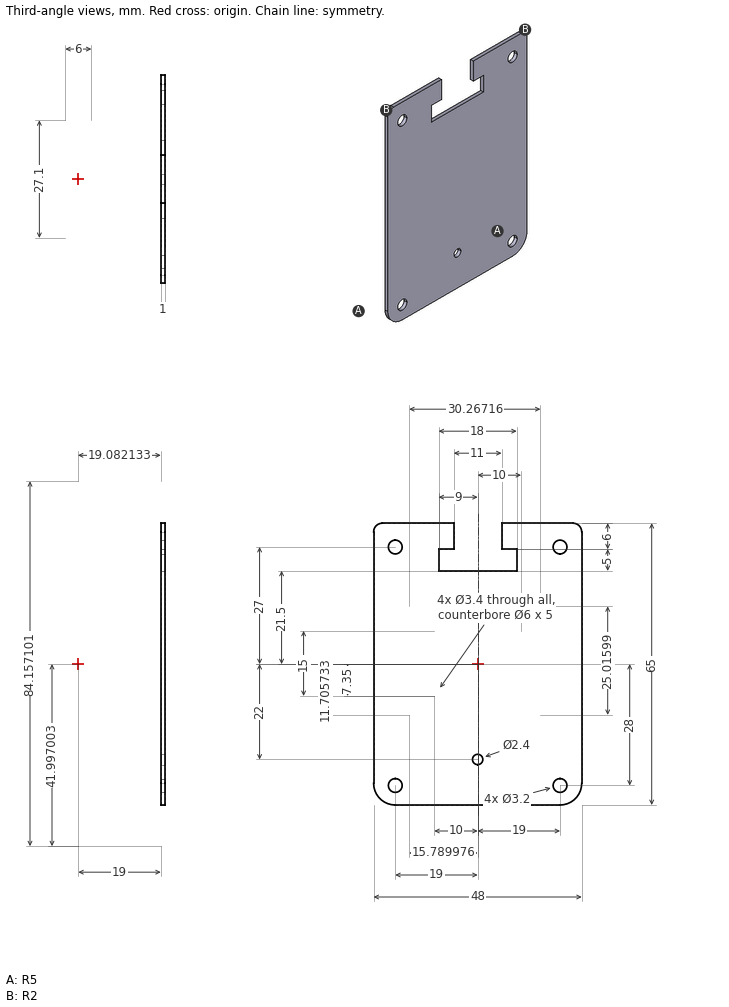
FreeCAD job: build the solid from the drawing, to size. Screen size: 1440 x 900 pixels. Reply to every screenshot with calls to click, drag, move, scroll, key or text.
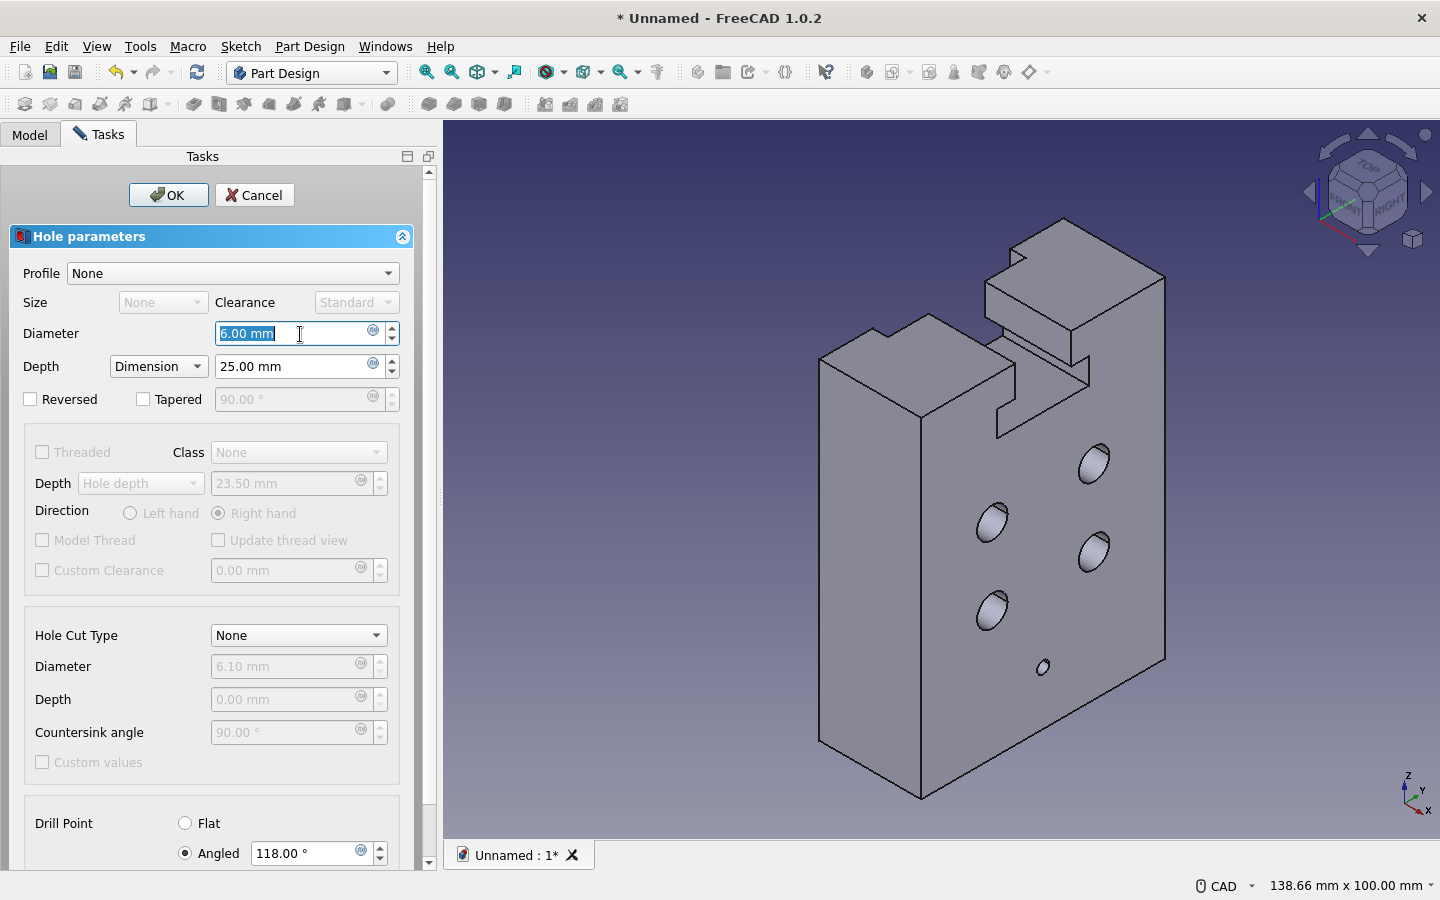
text(3.4)
key(Tab)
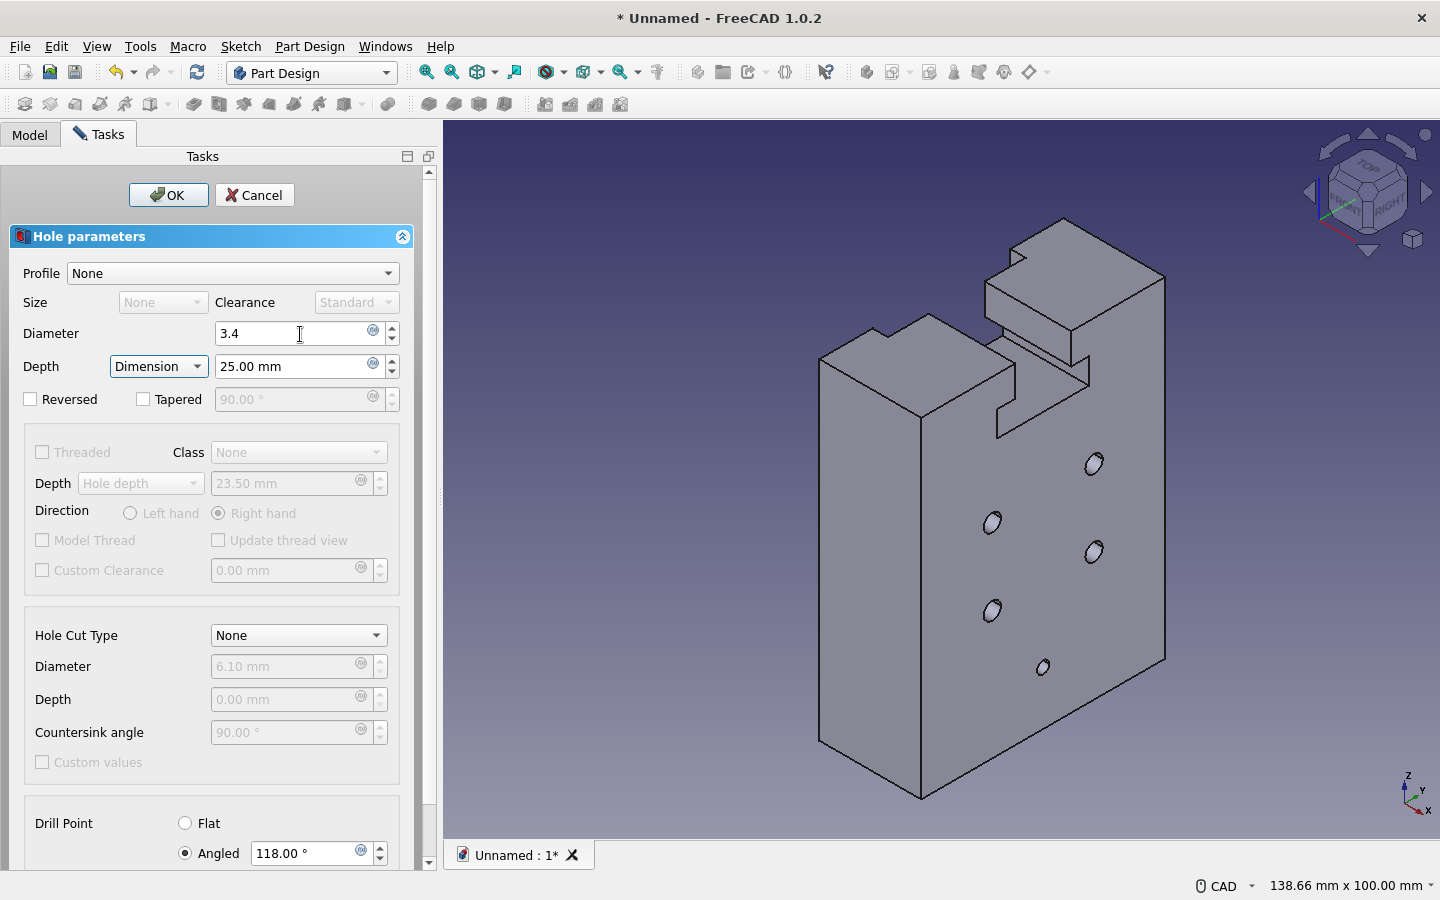
click(160, 366)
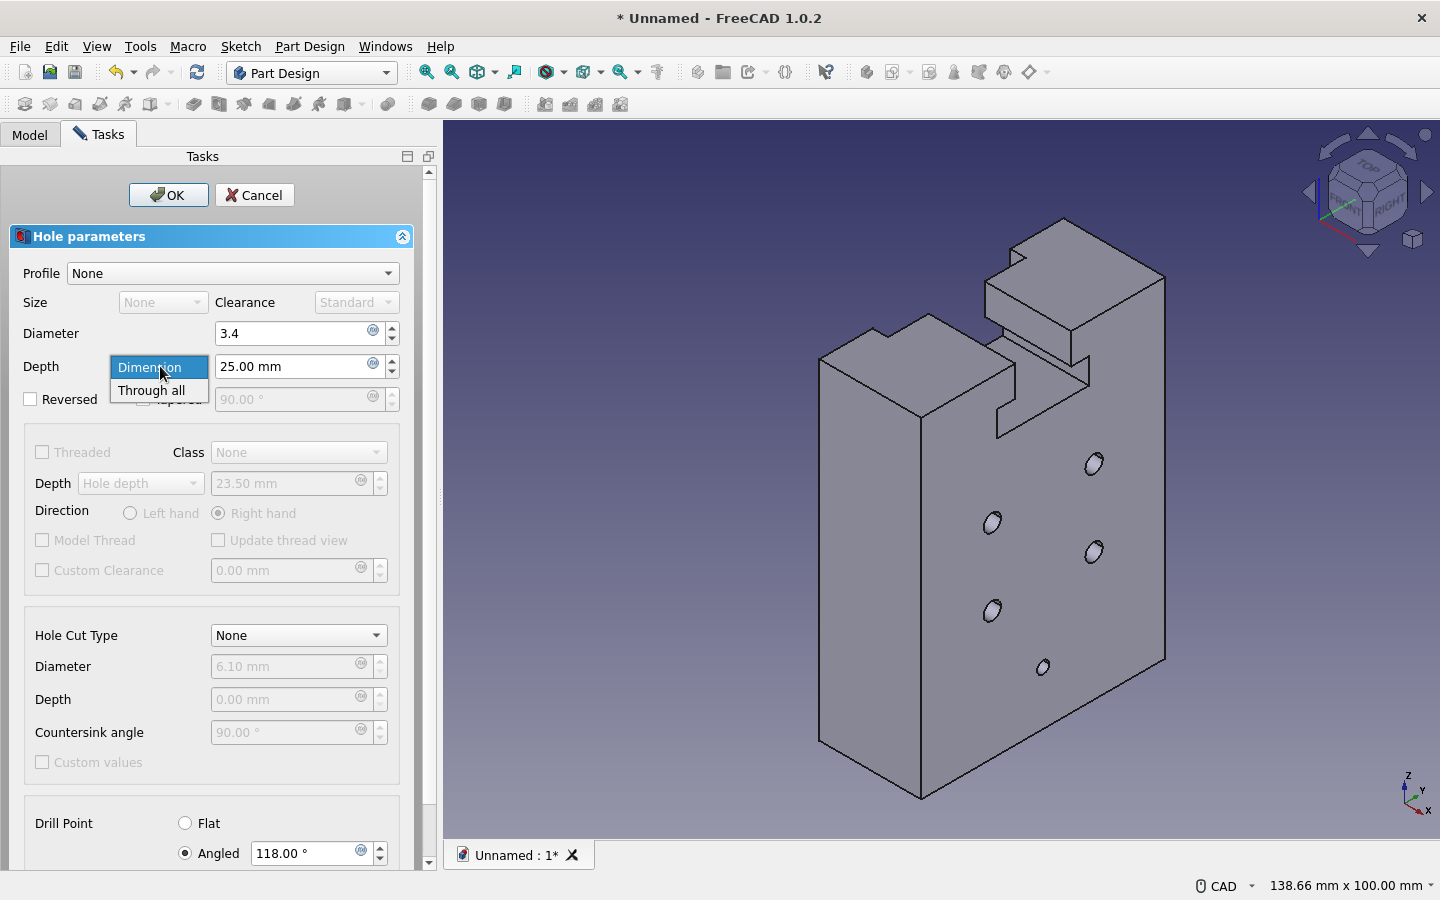
click(158, 390)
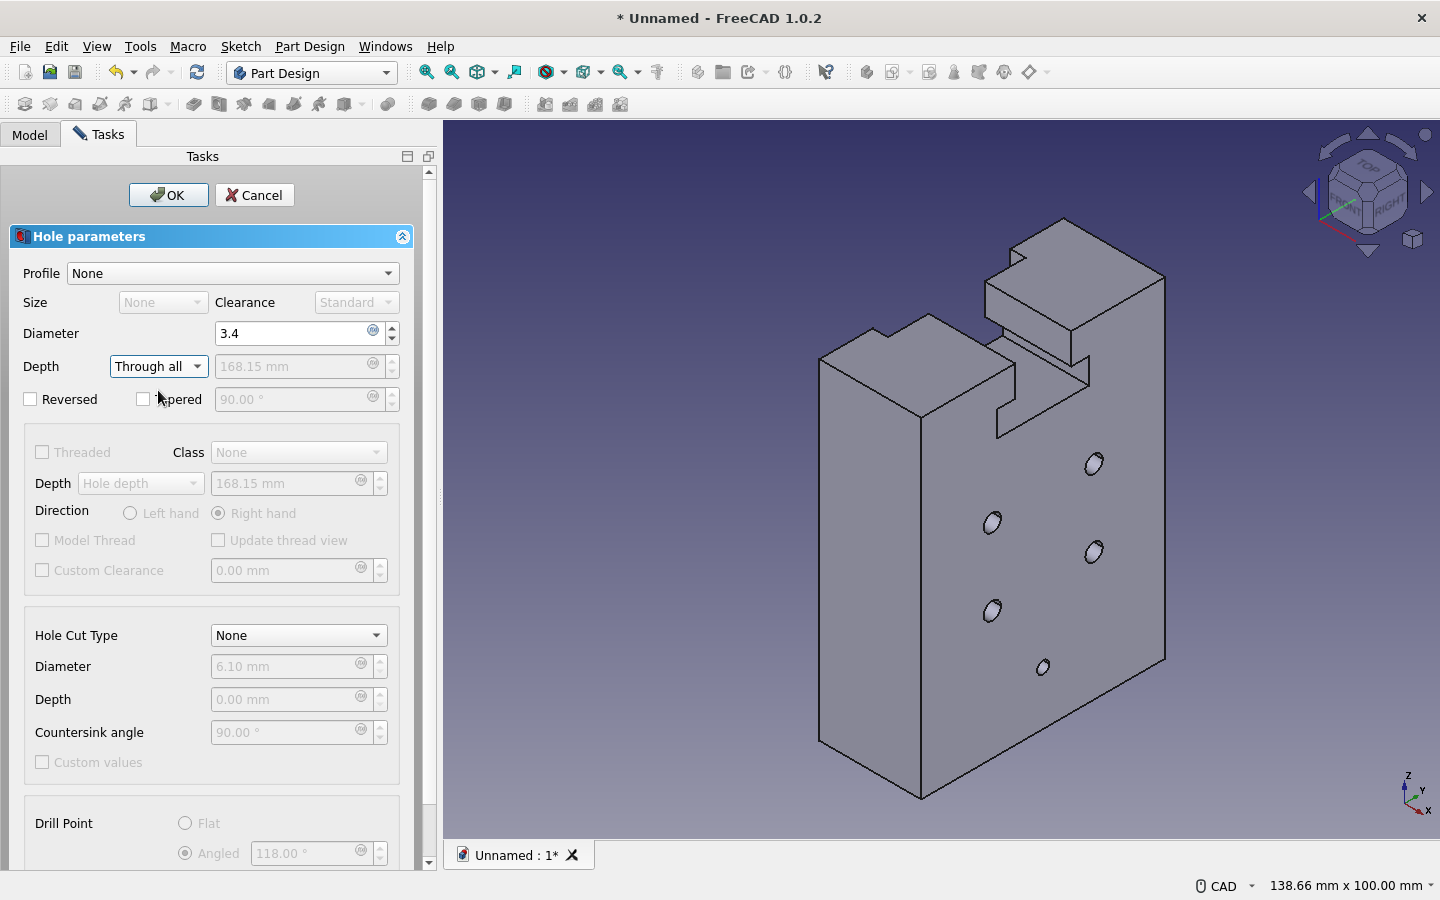
click(300, 636)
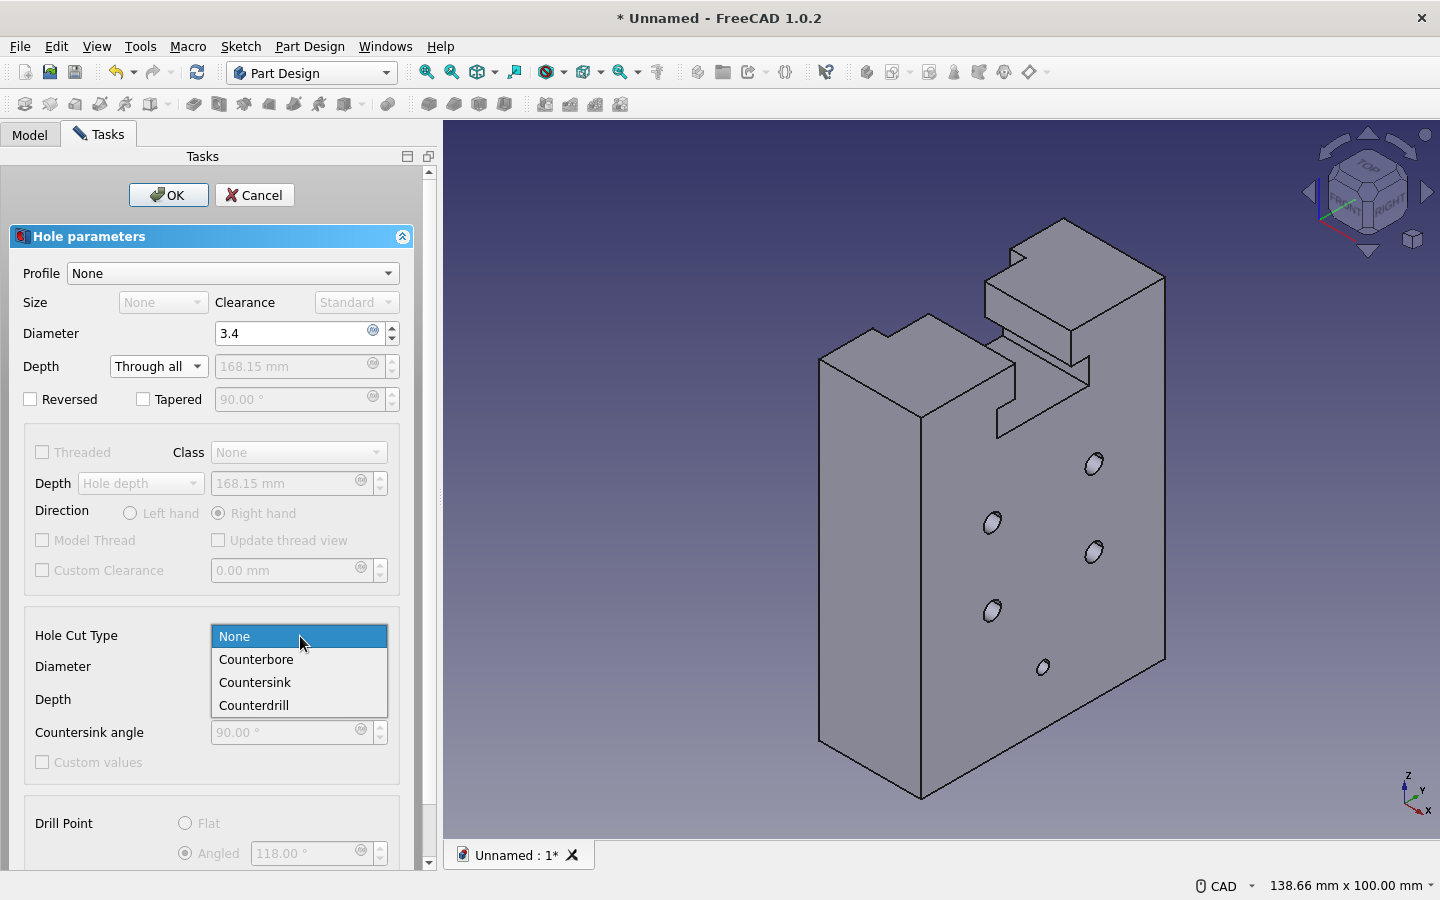
click(298, 660)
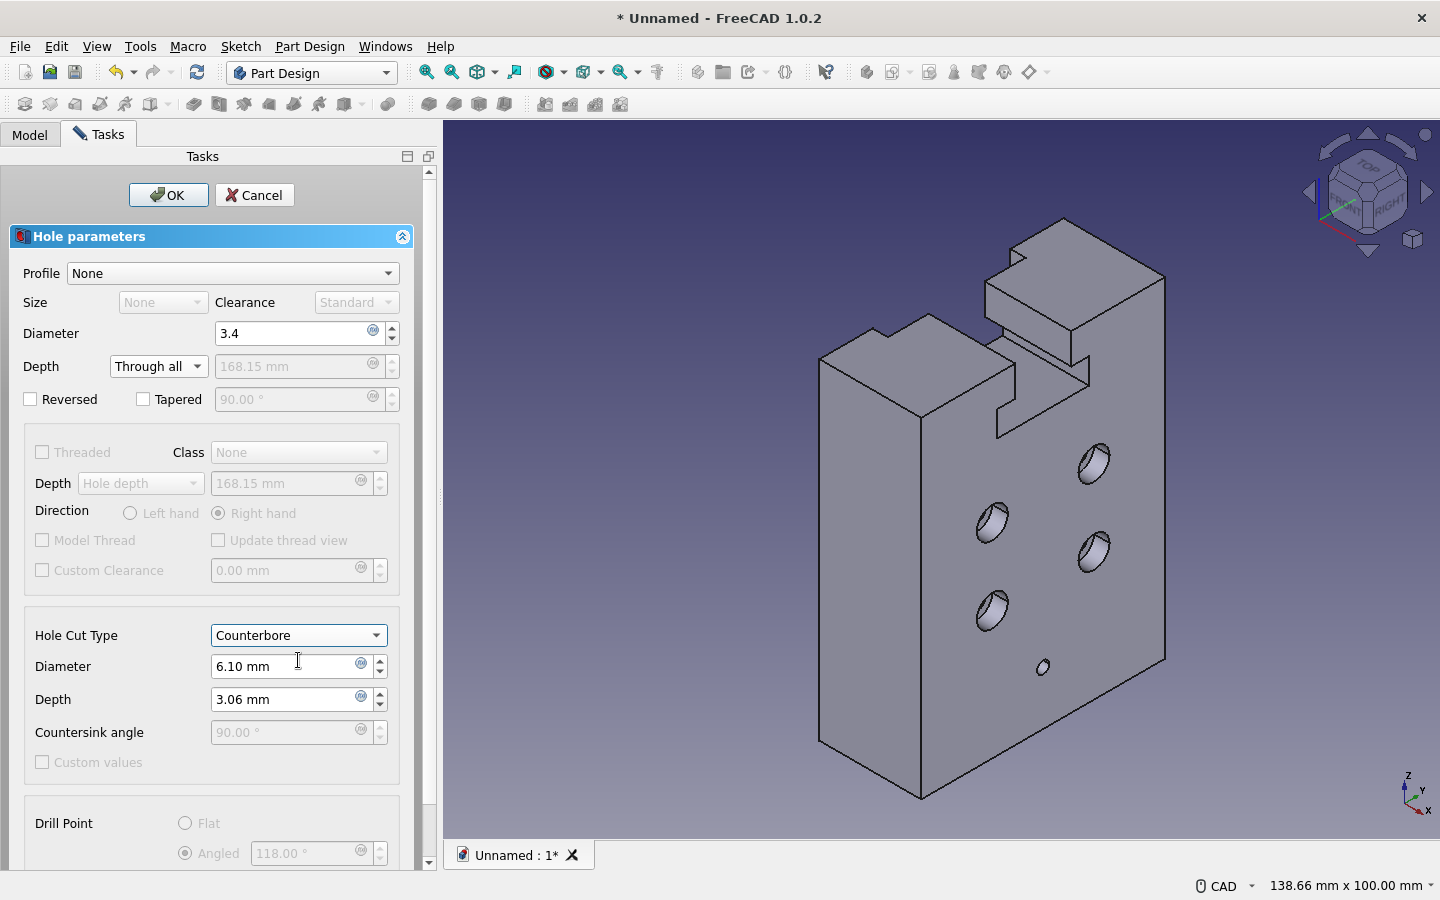
triple_click(292, 666)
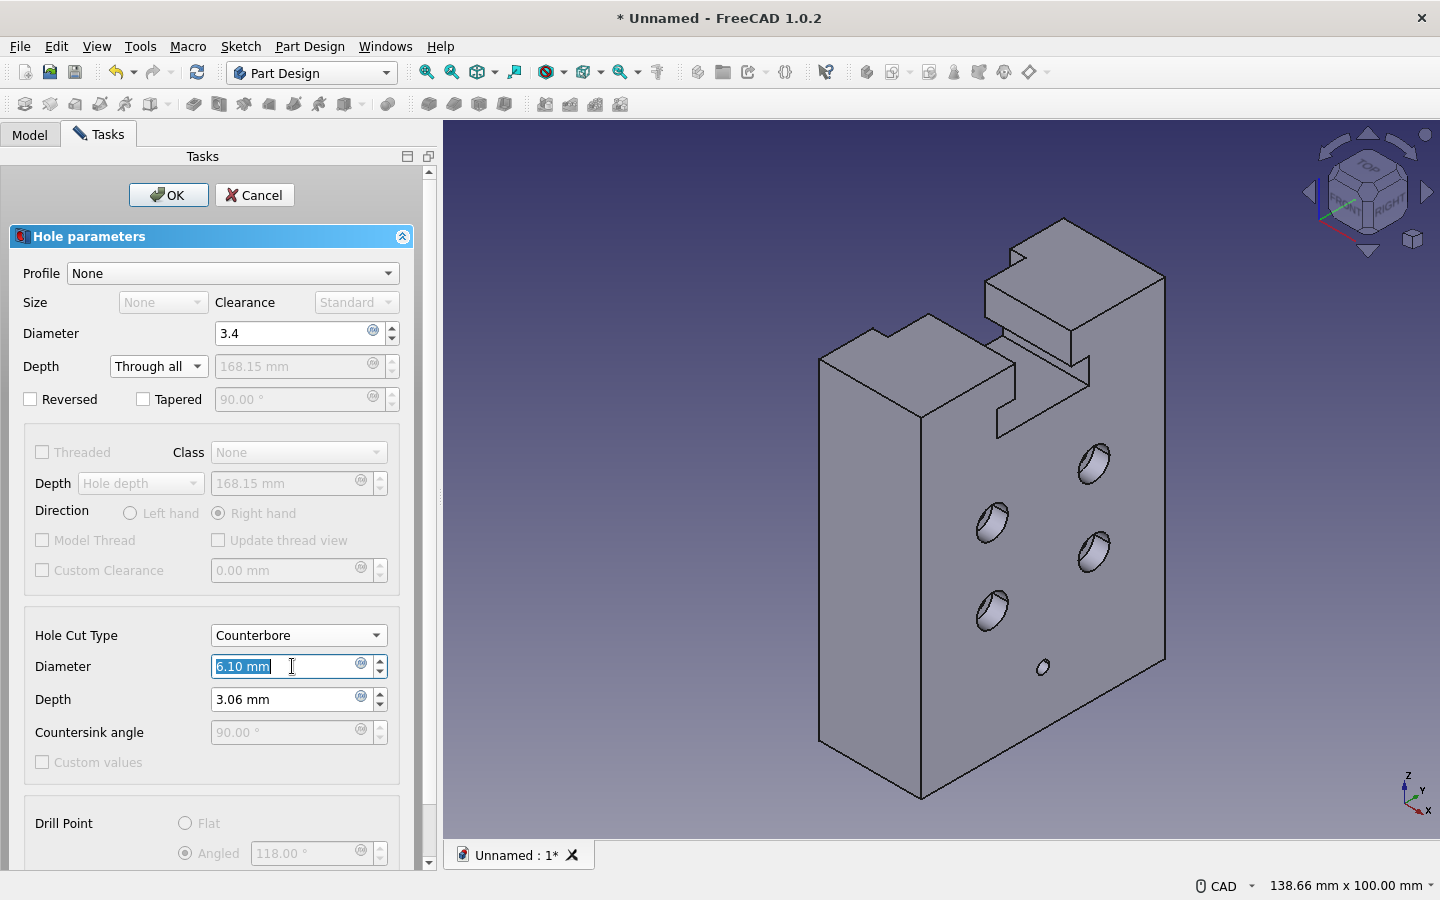
text(6)
key(Tab)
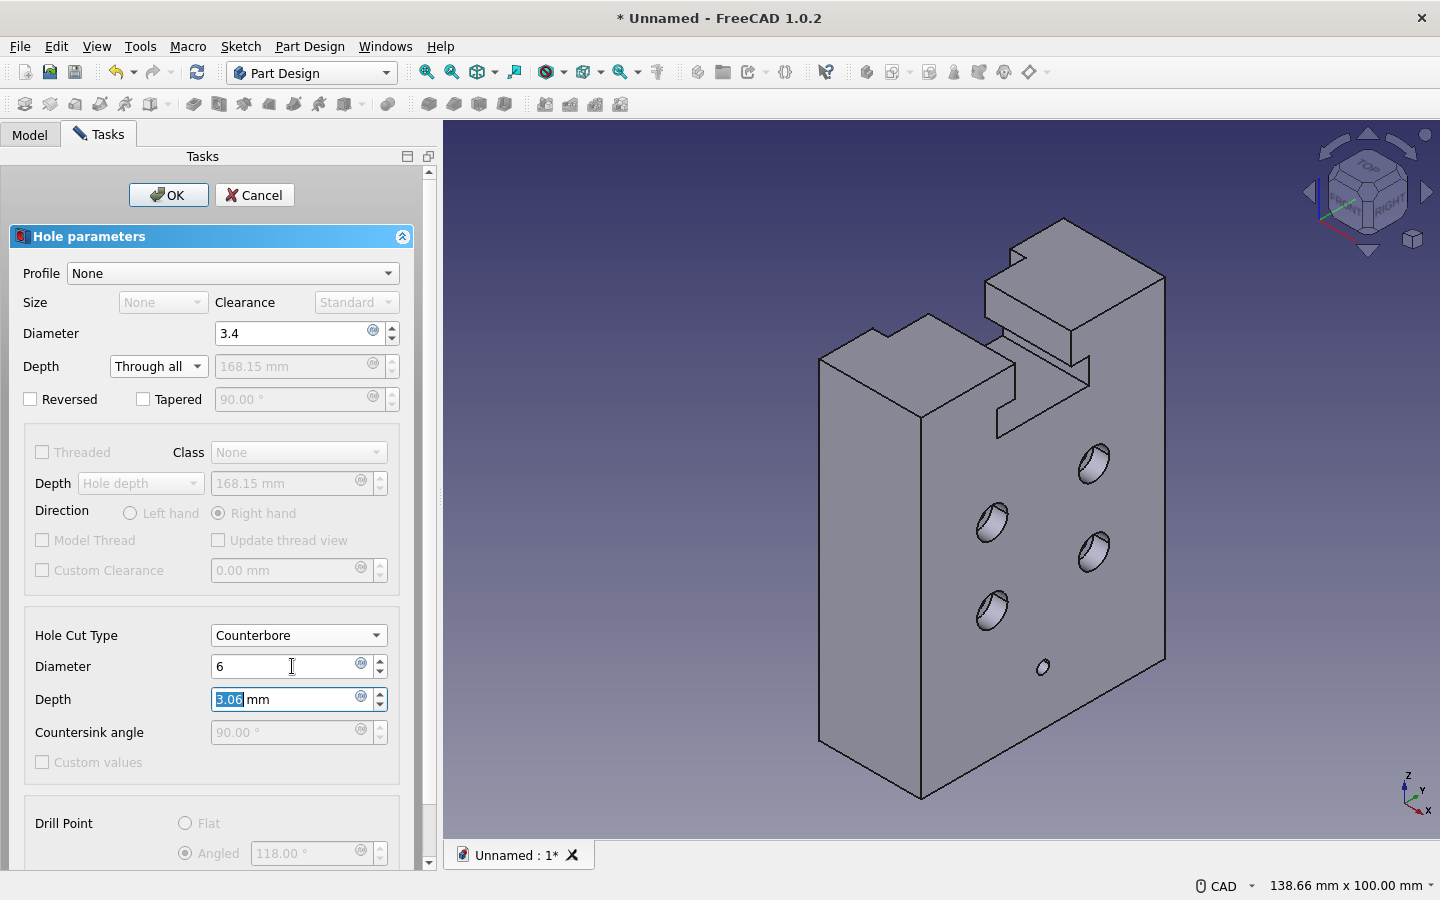
text(5)
key(Tab)